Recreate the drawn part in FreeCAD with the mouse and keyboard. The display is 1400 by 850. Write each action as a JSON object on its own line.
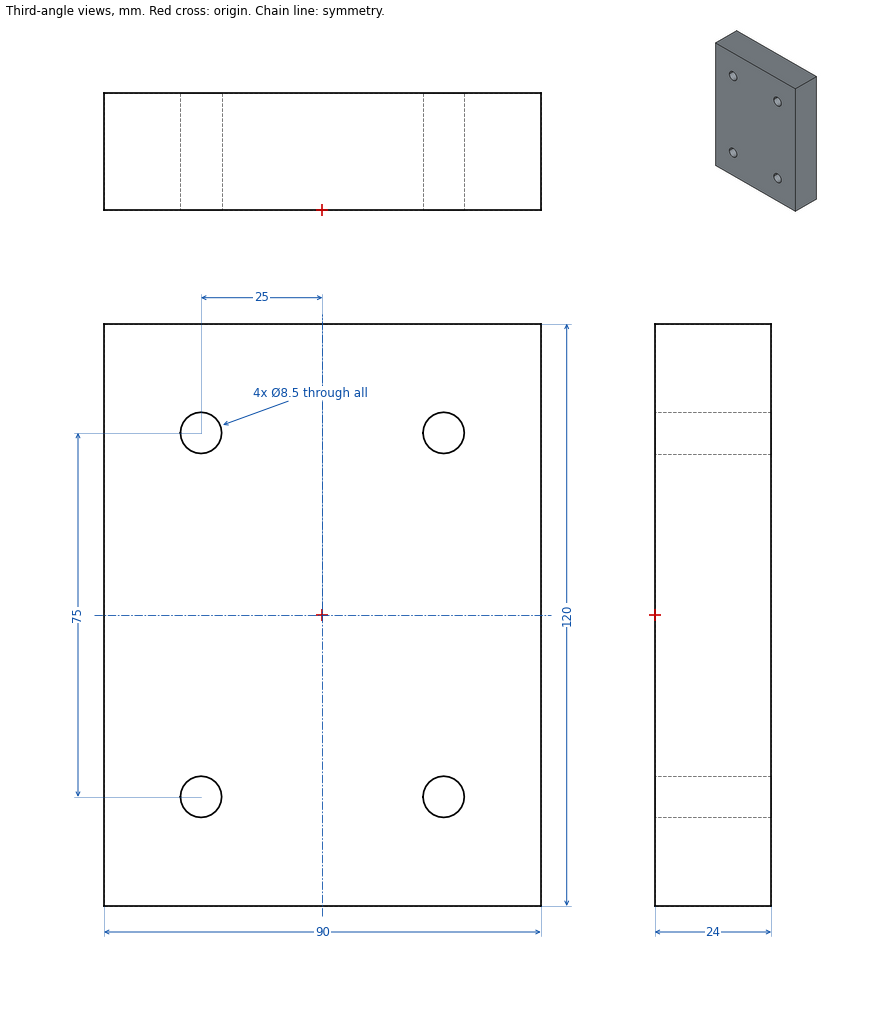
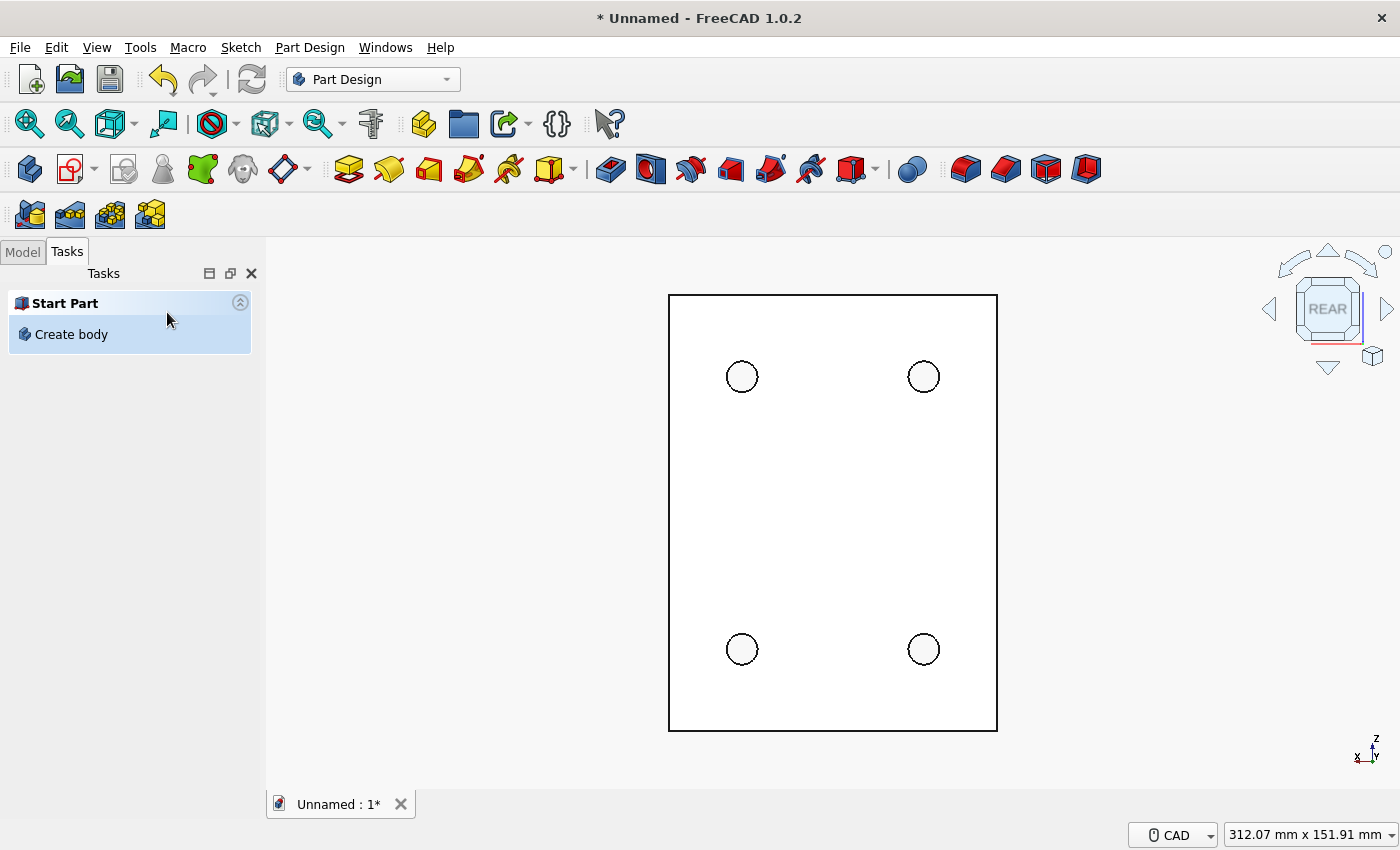
{"action": "key", "text": "0"}